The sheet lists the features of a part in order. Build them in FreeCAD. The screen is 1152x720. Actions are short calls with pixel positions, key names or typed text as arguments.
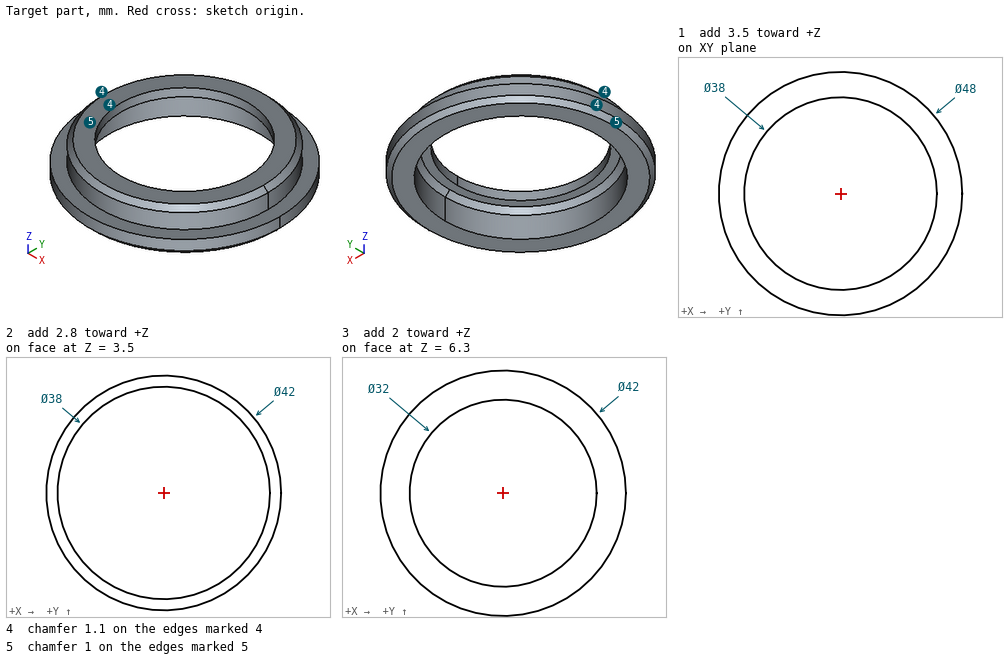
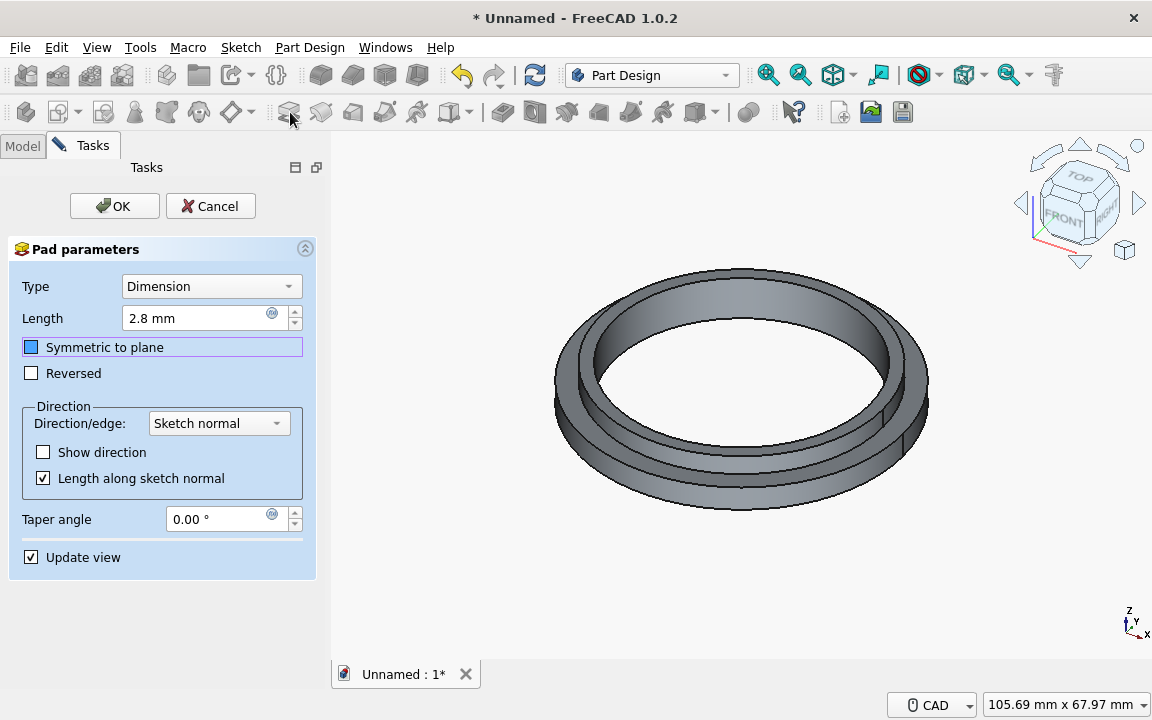
click(115, 206)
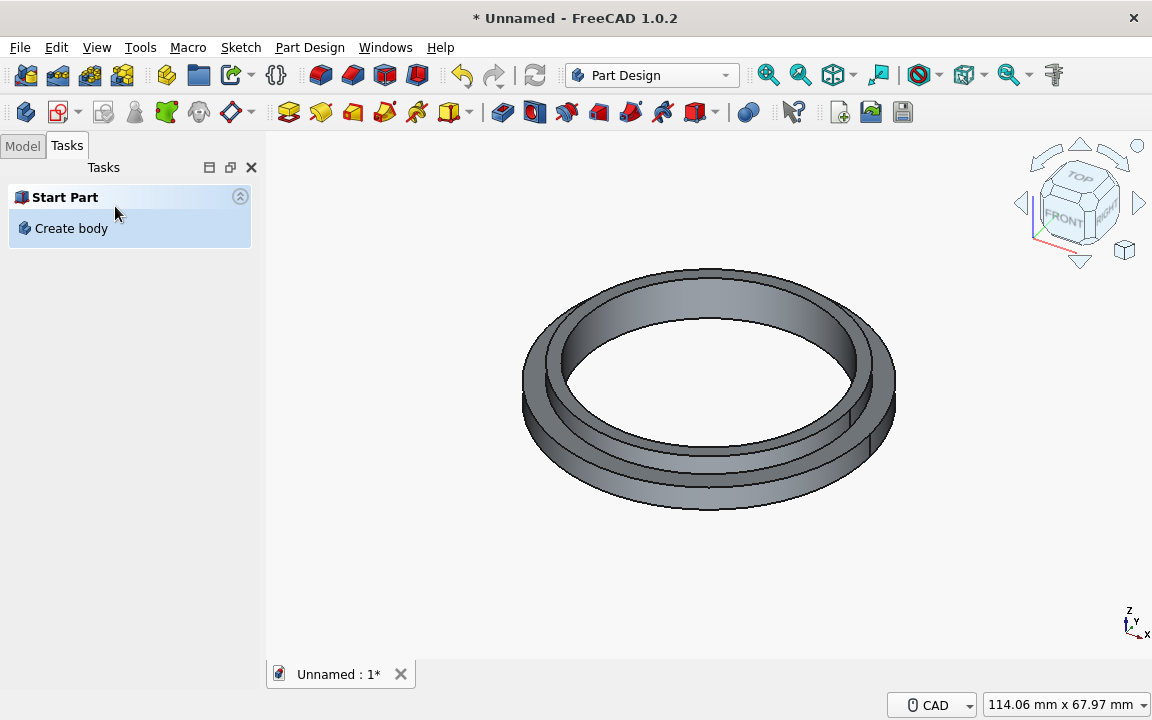
scroll(864, 380, up, 5)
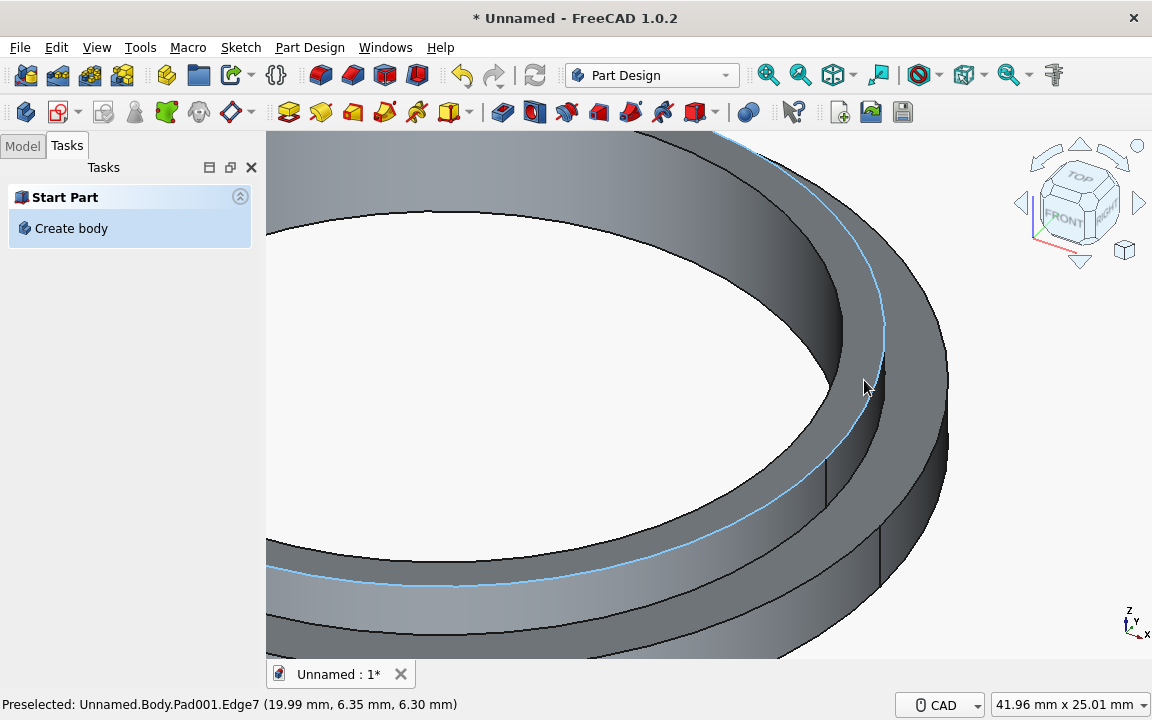
click(862, 382)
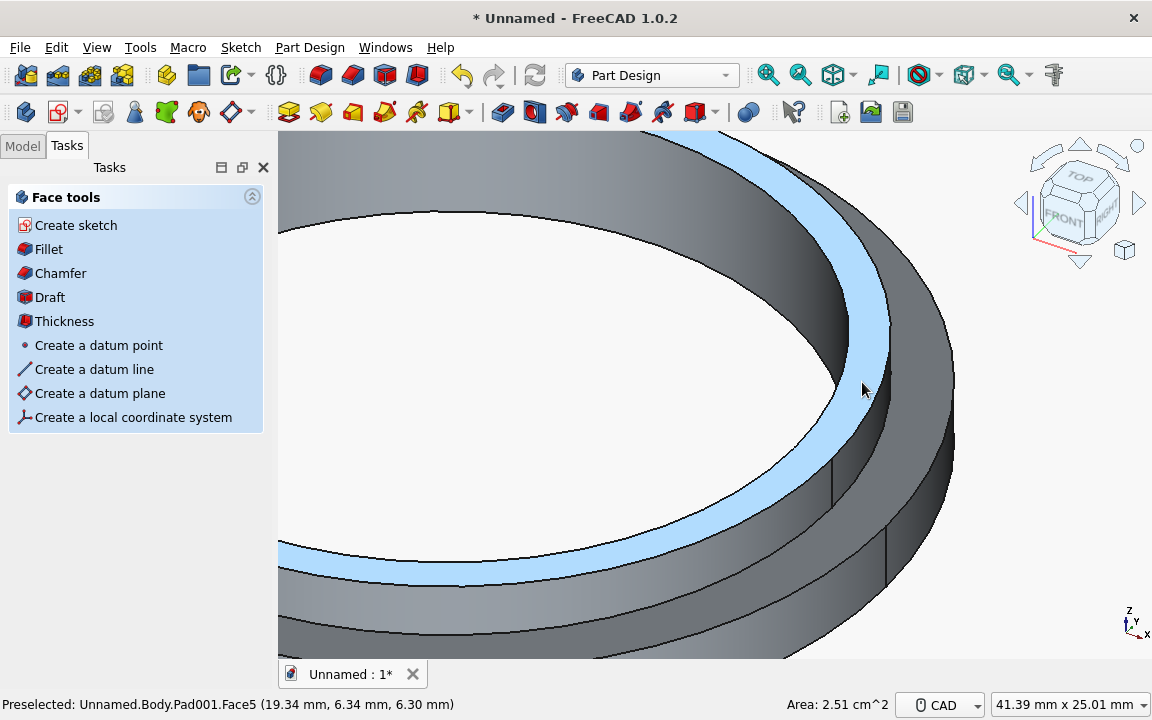
click(58, 112)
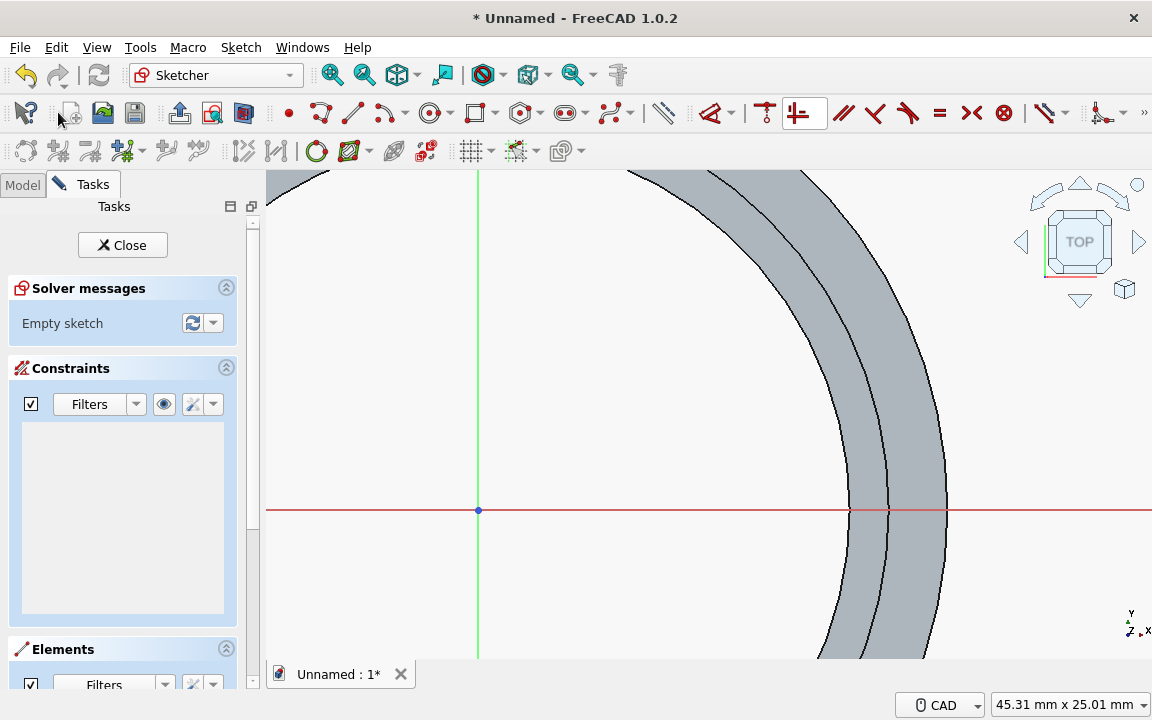
scroll(735, 359, down, 5)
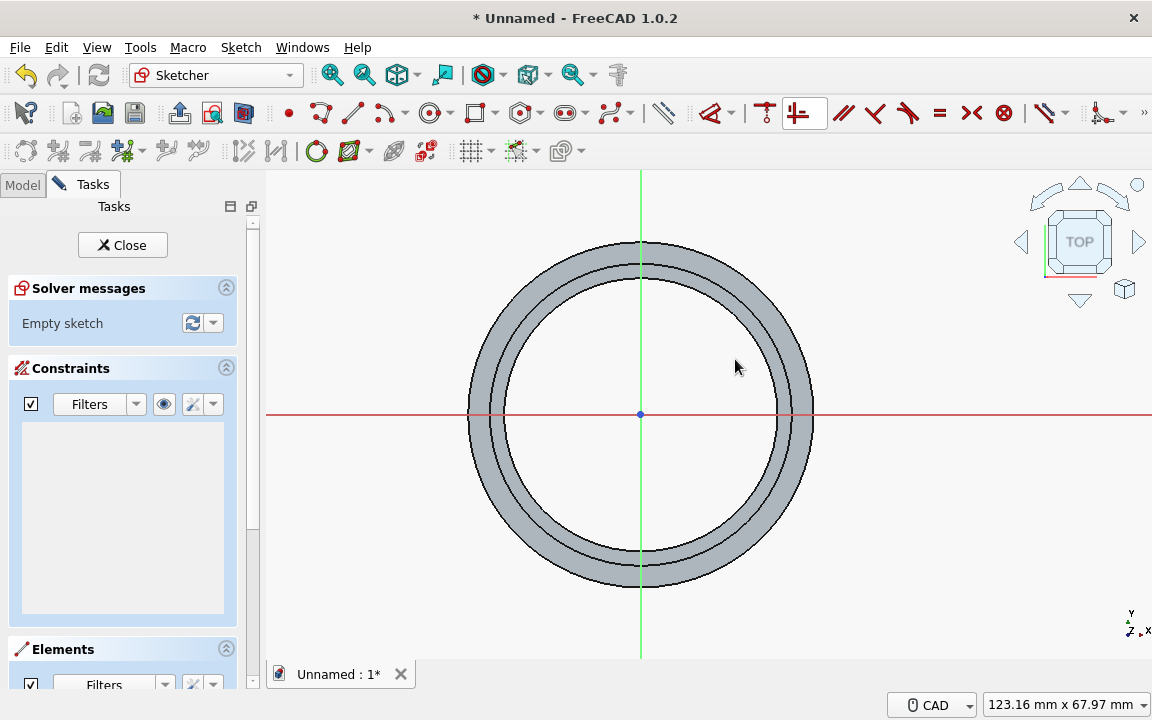
click(430, 114)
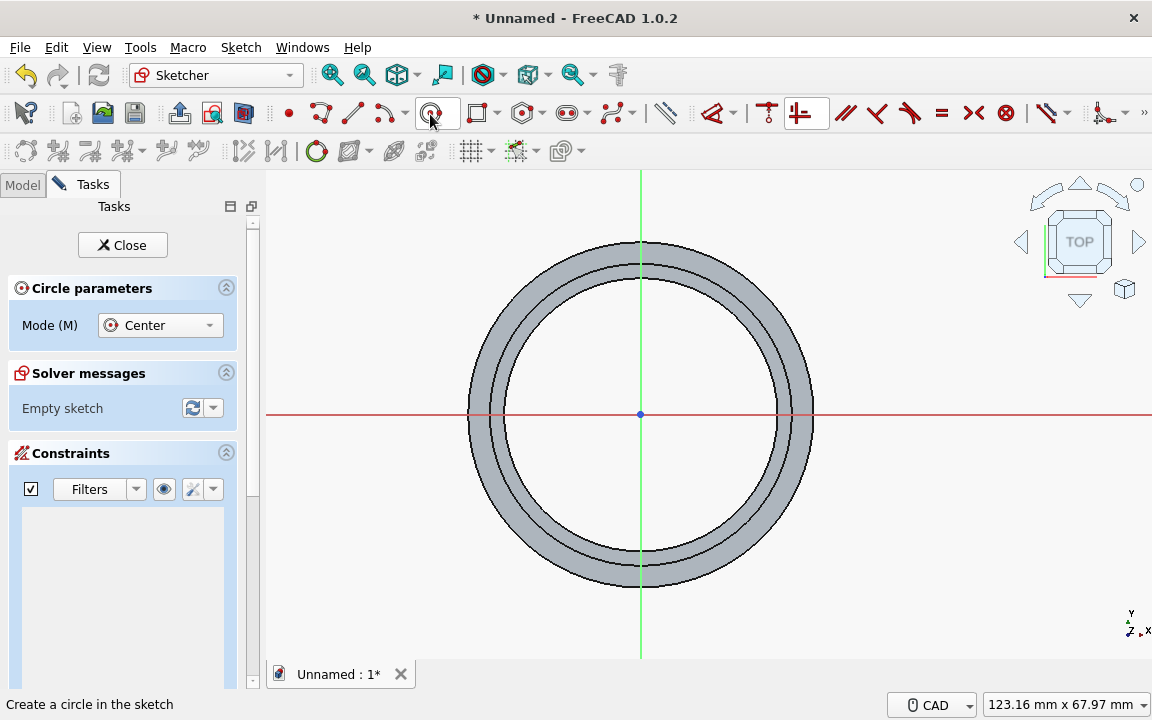
click(641, 415)
move(748, 308)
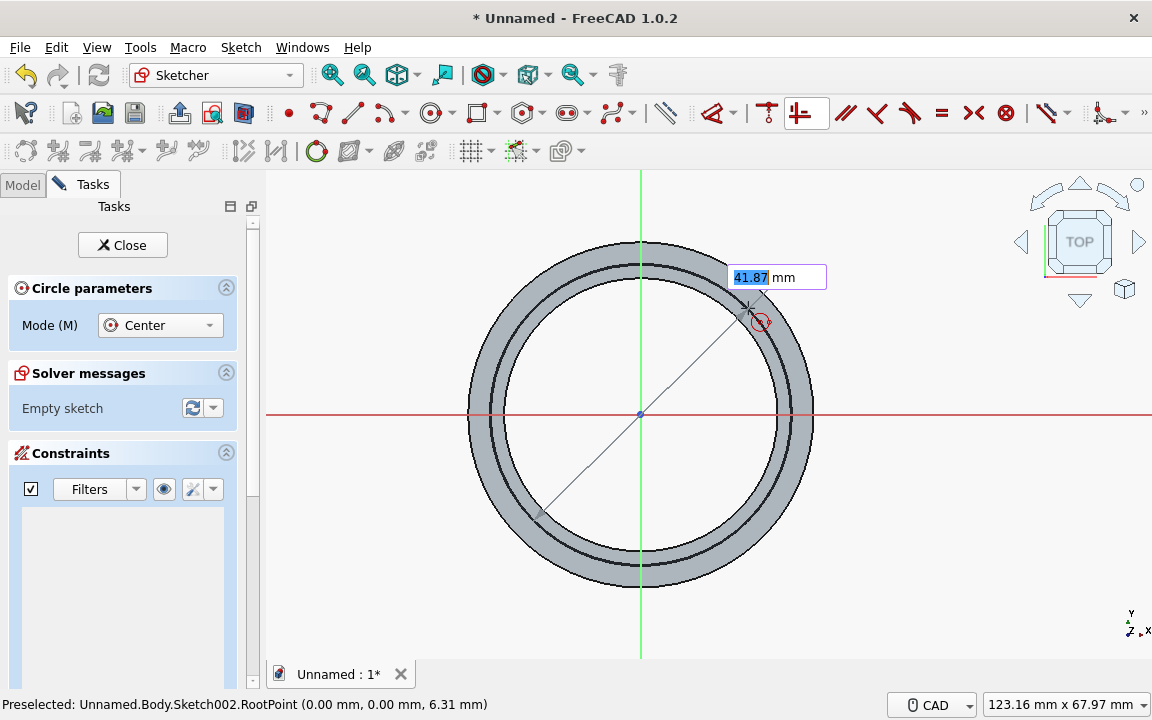
text(42)
key(Return)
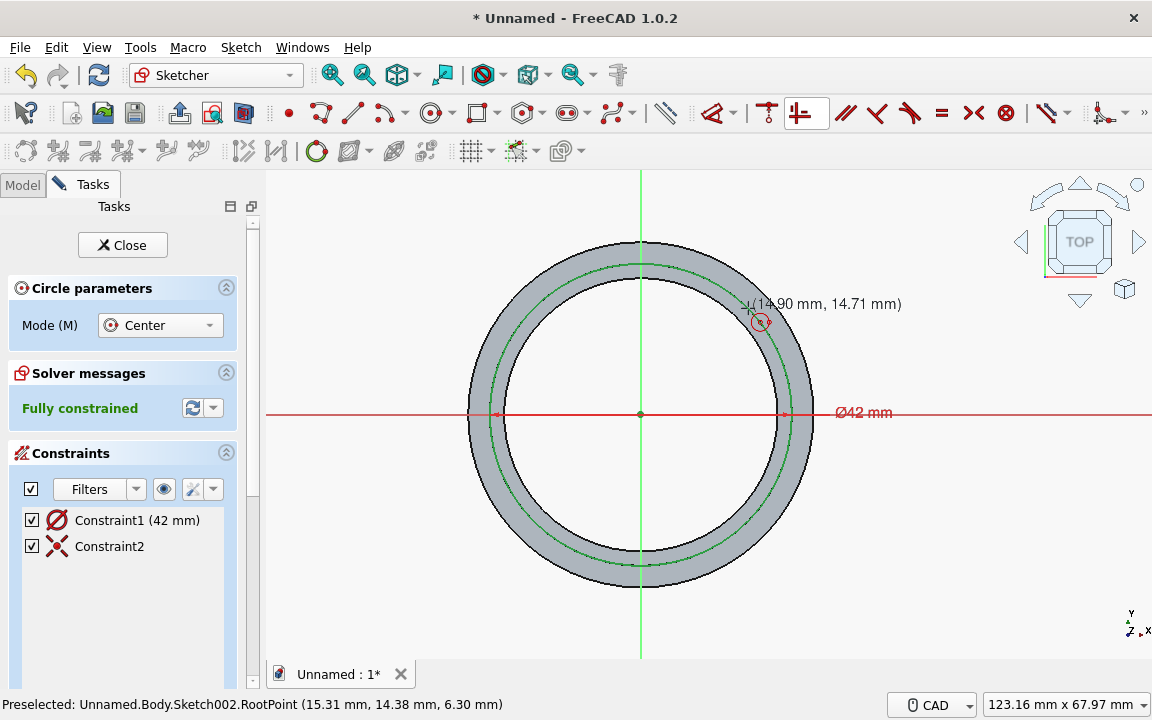
click(641, 415)
move(722, 333)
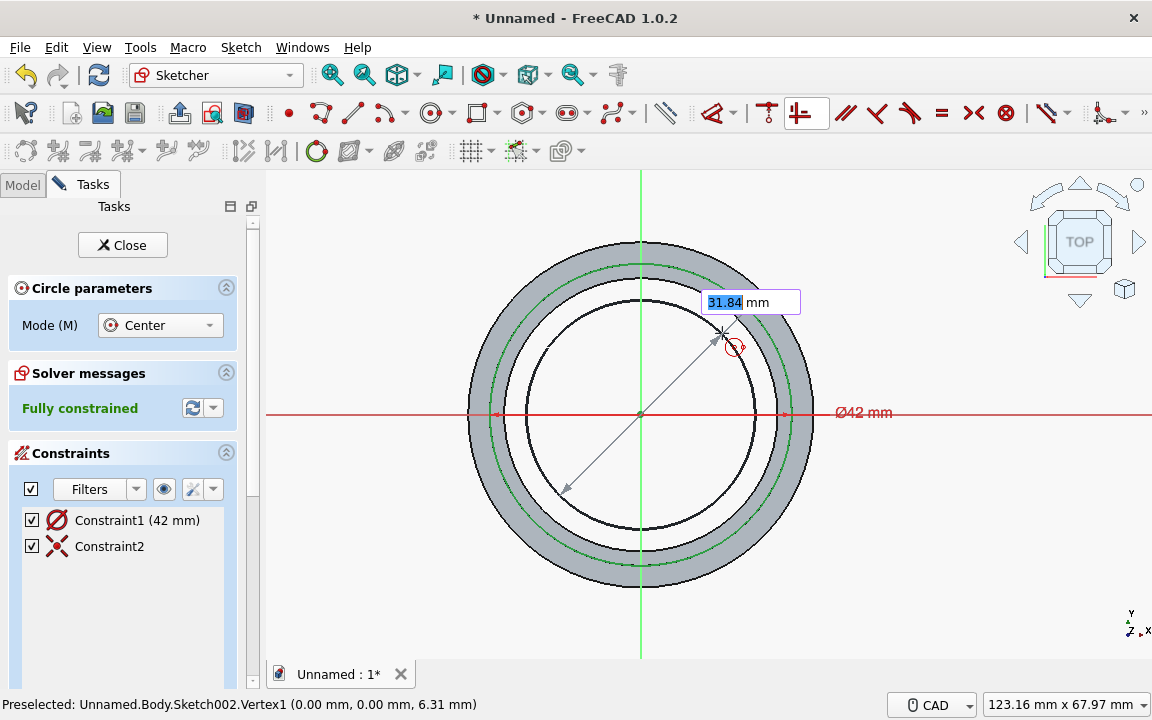
text(32)
key(Return)
key(Escape)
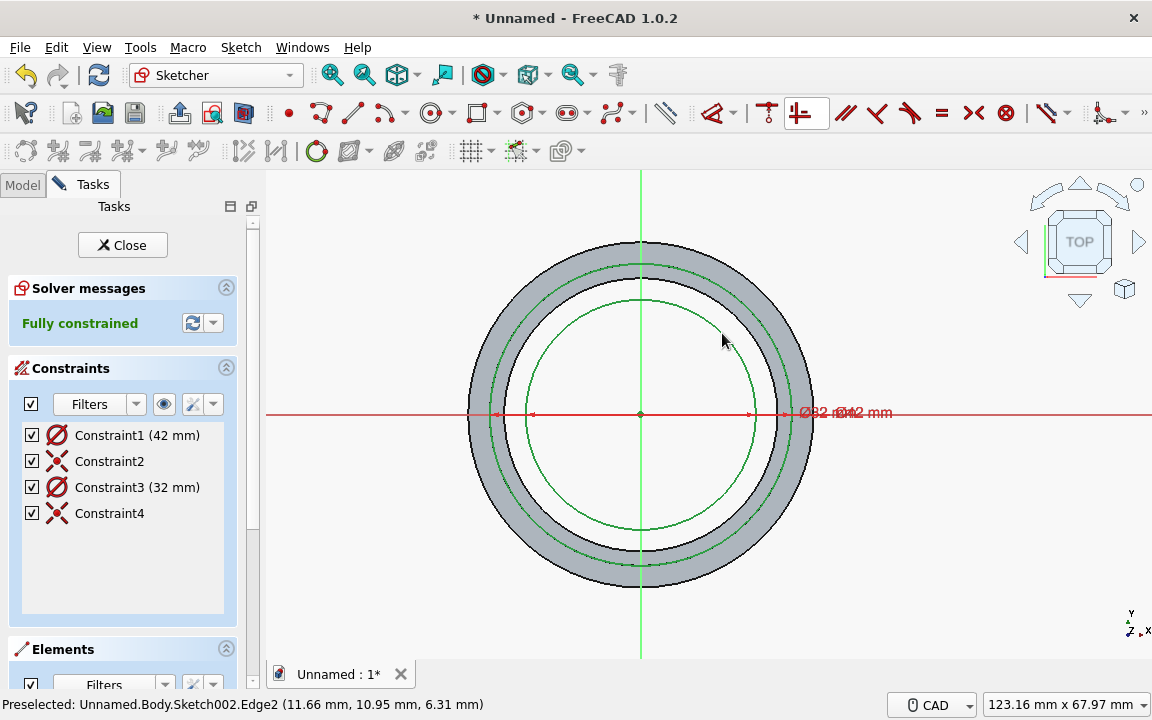
click(123, 245)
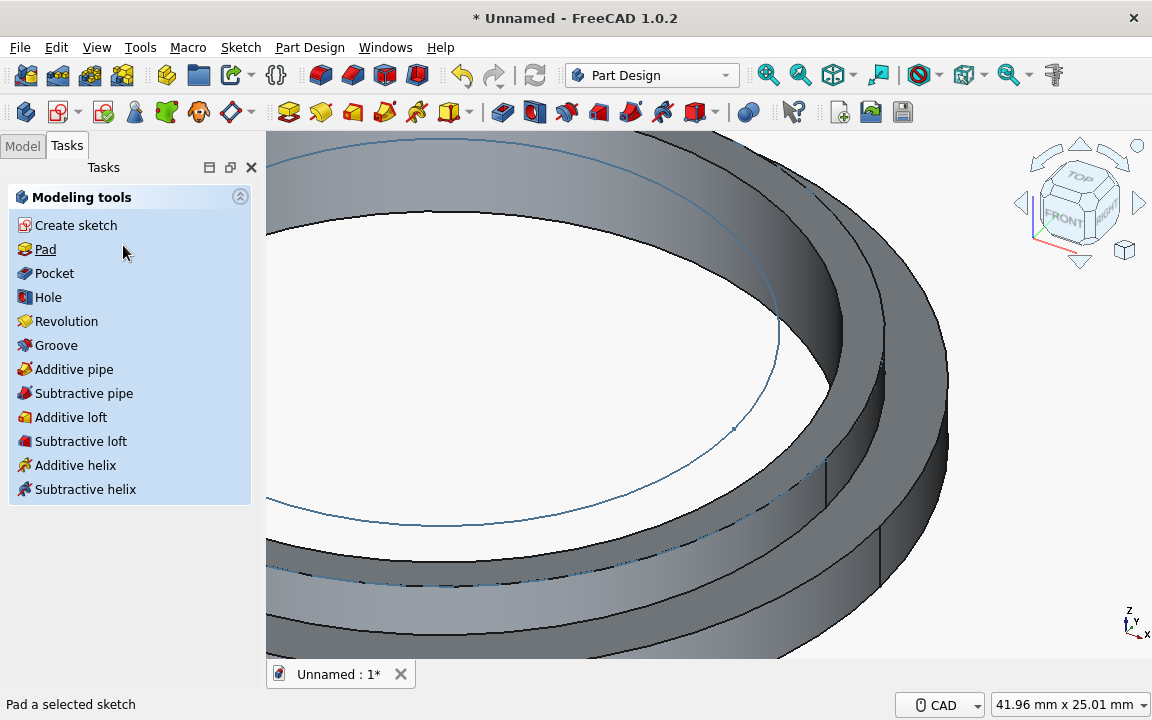
click(290, 112)